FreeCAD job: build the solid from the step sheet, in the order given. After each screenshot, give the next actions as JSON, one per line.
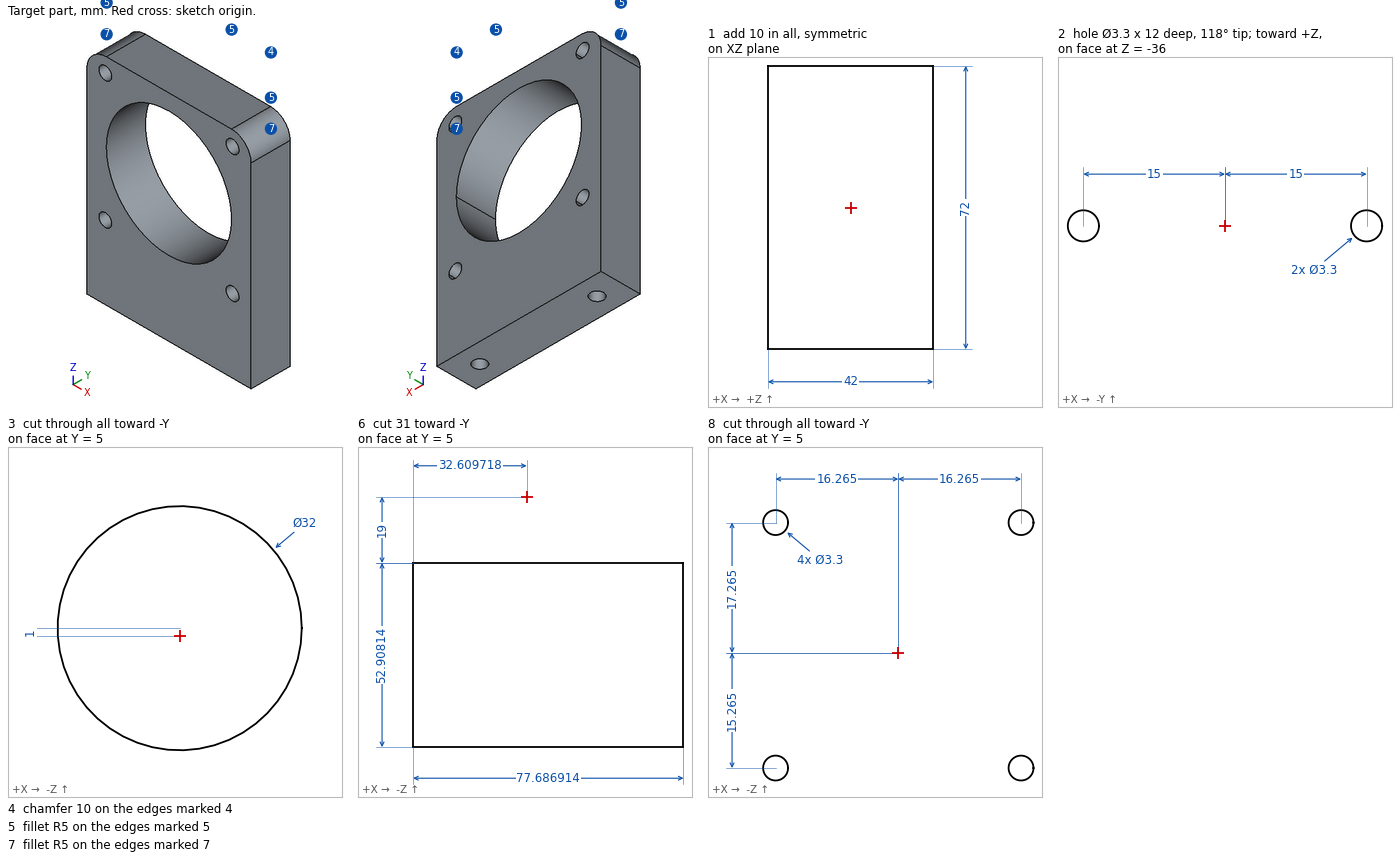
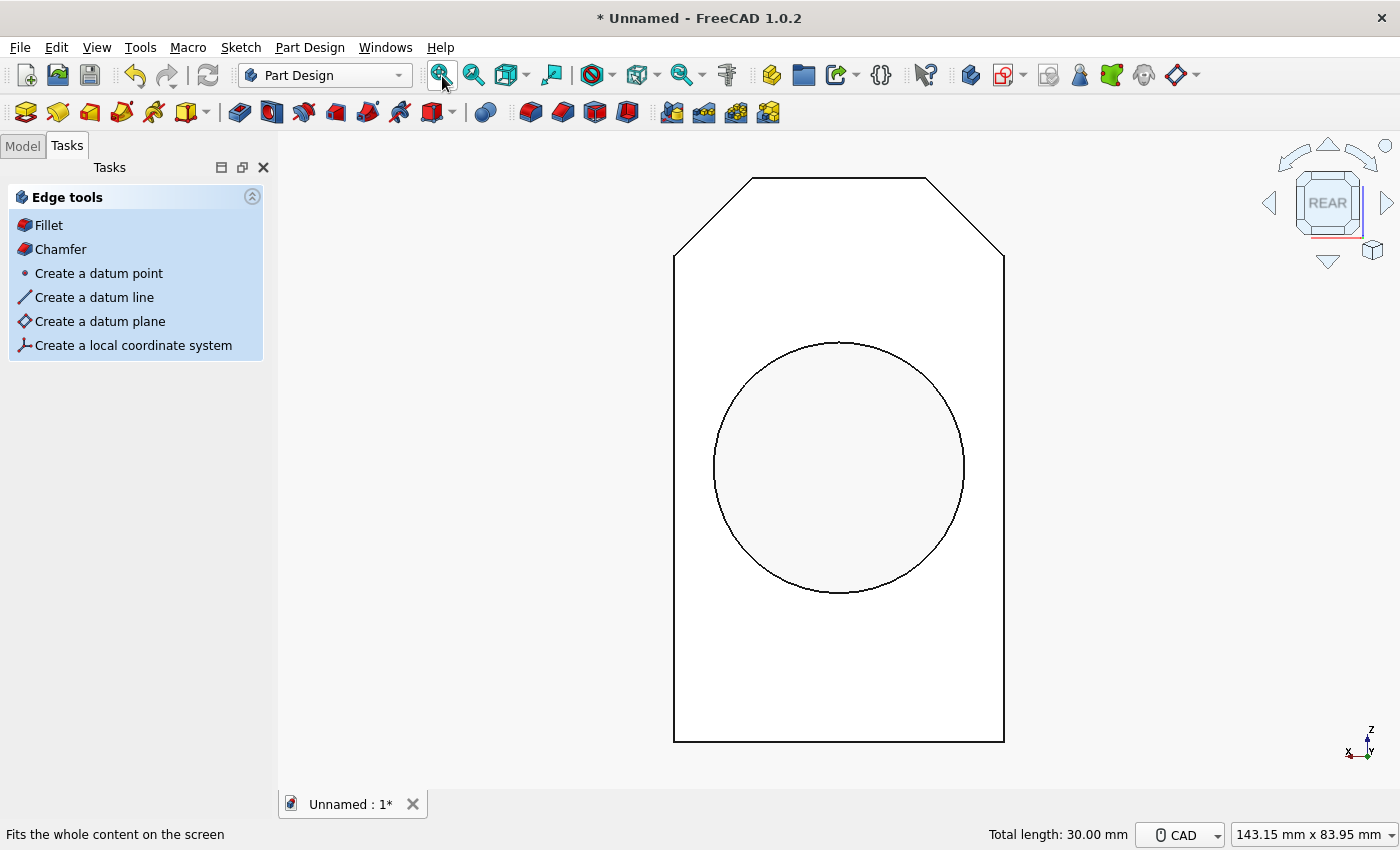
{"action": "key", "text": "6"}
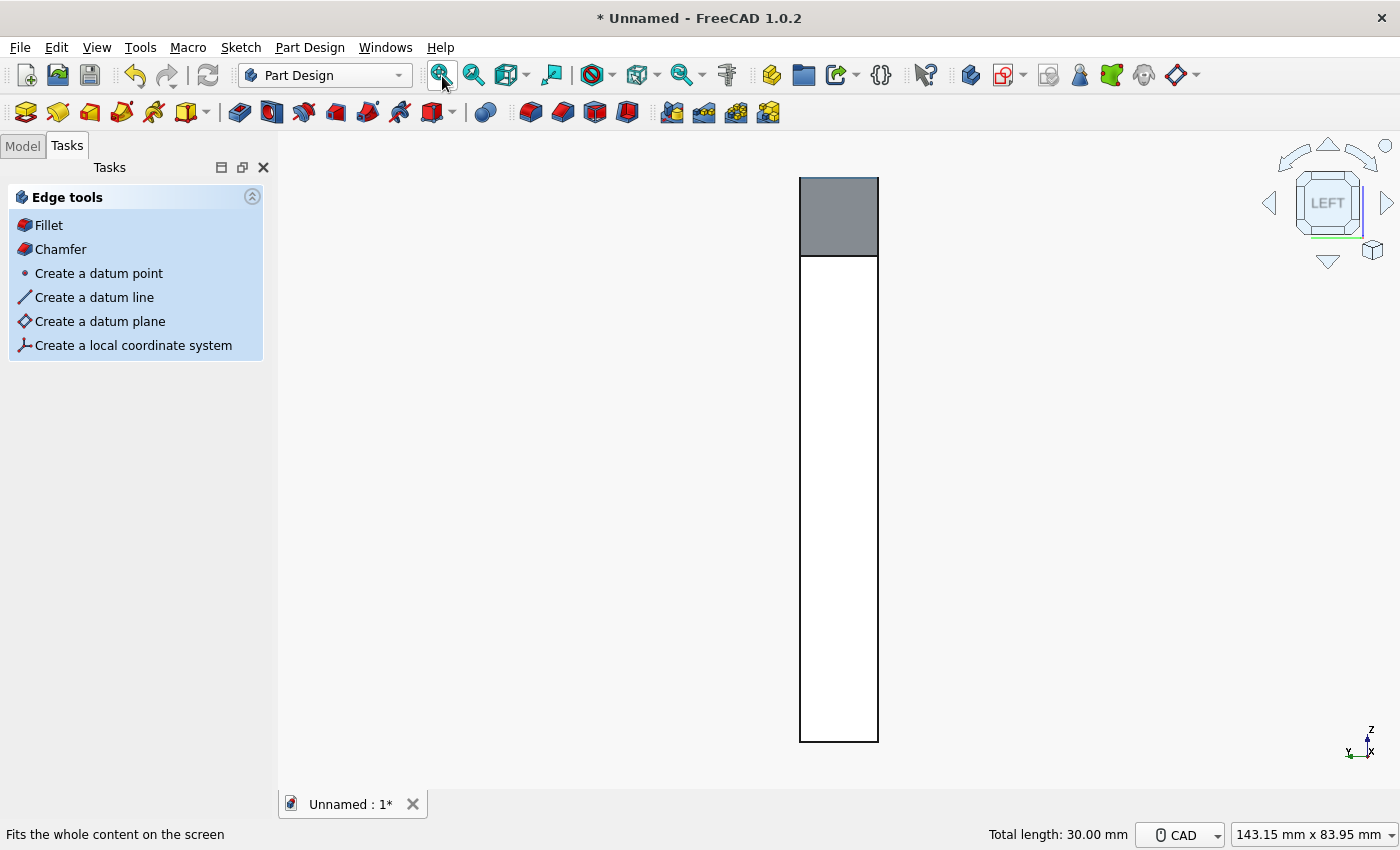
{"action": "left_click", "coordinate": [839, 255], "text": "ctrl"}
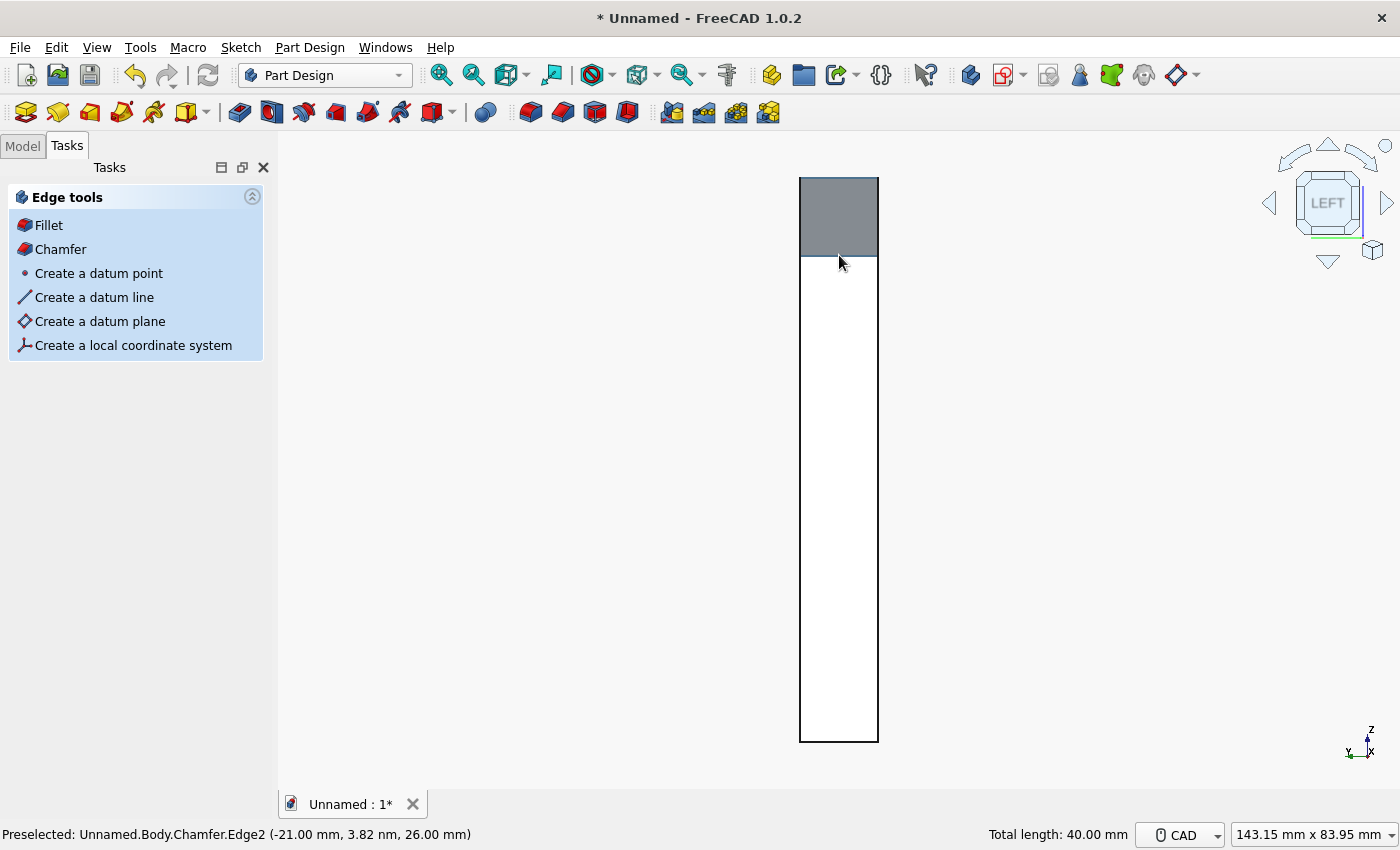
{"action": "left_click", "coordinate": [532, 112]}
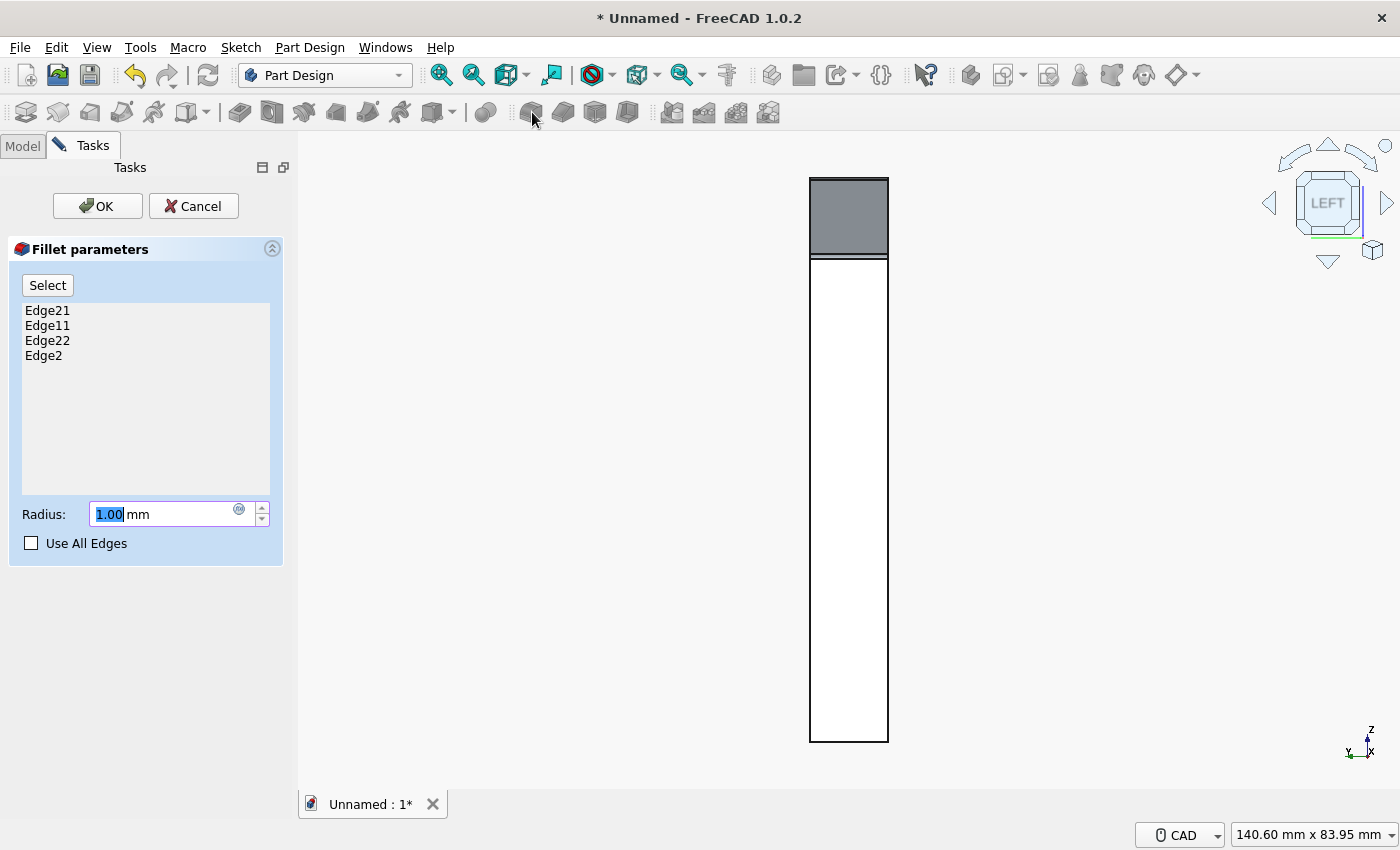
{"action": "type", "text": "5"}
{"action": "key", "text": "Tab"}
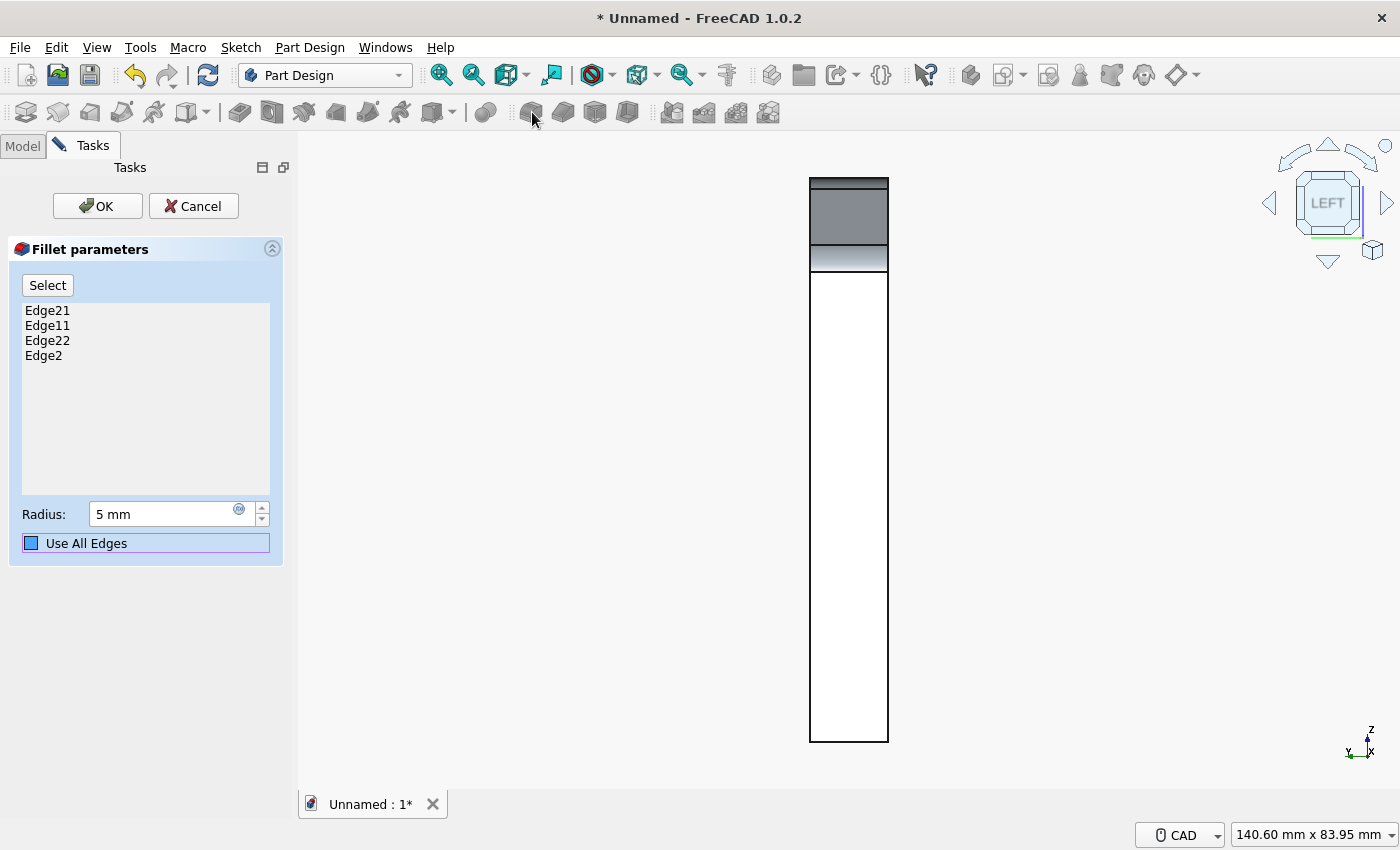
{"action": "left_click", "coordinate": [98, 206]}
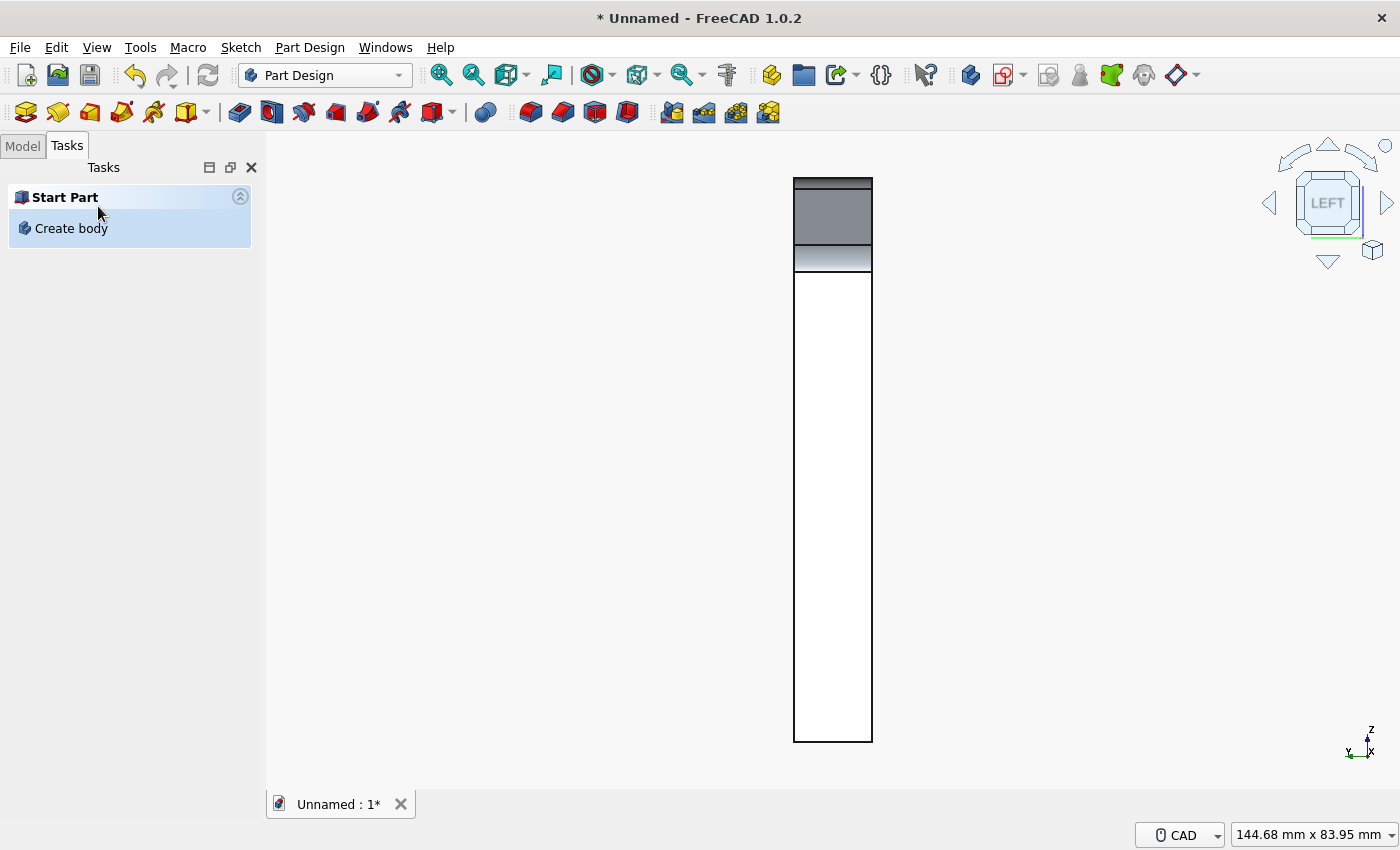
{"action": "key", "text": "4"}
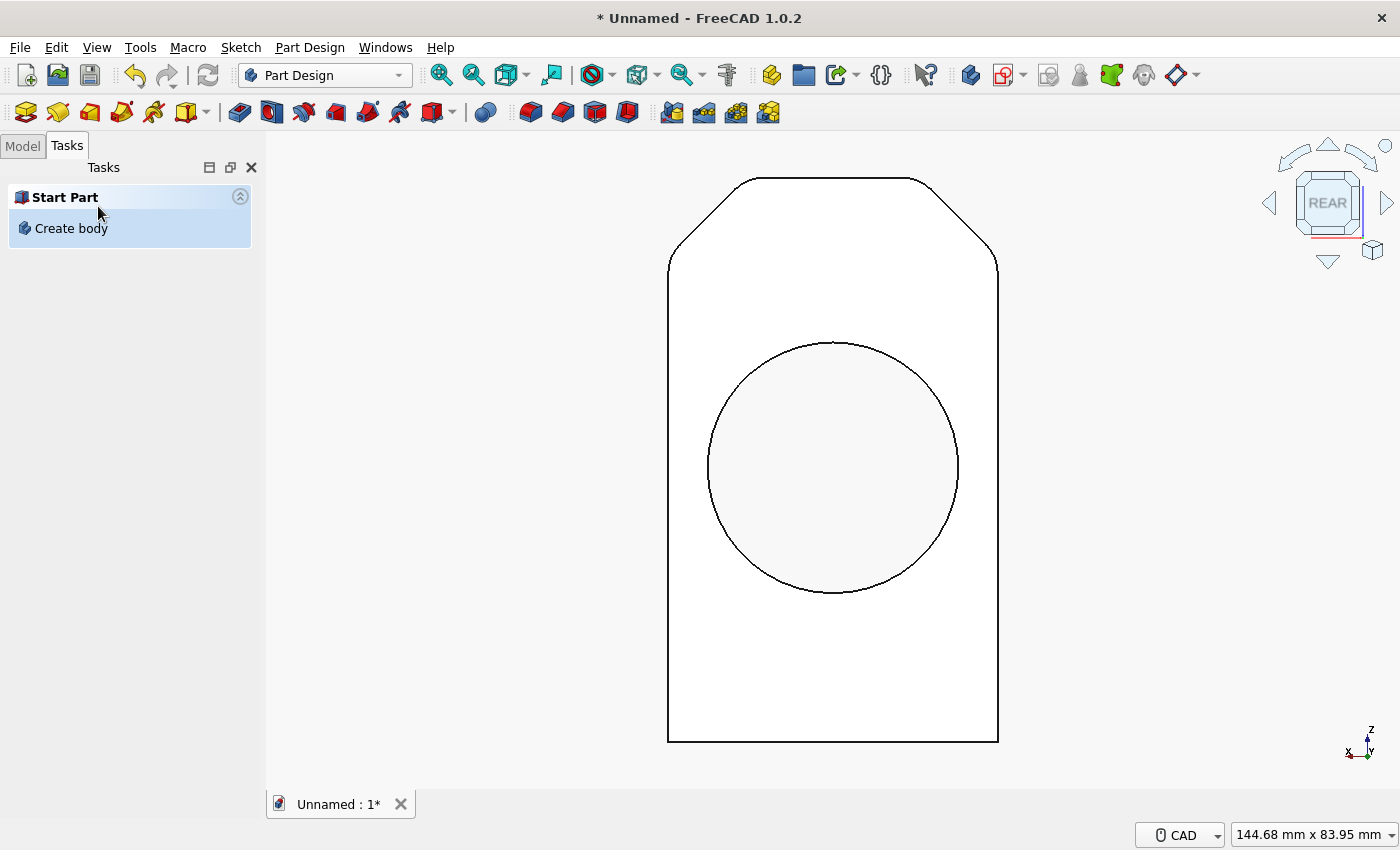
{"action": "left_click", "coordinate": [927, 298]}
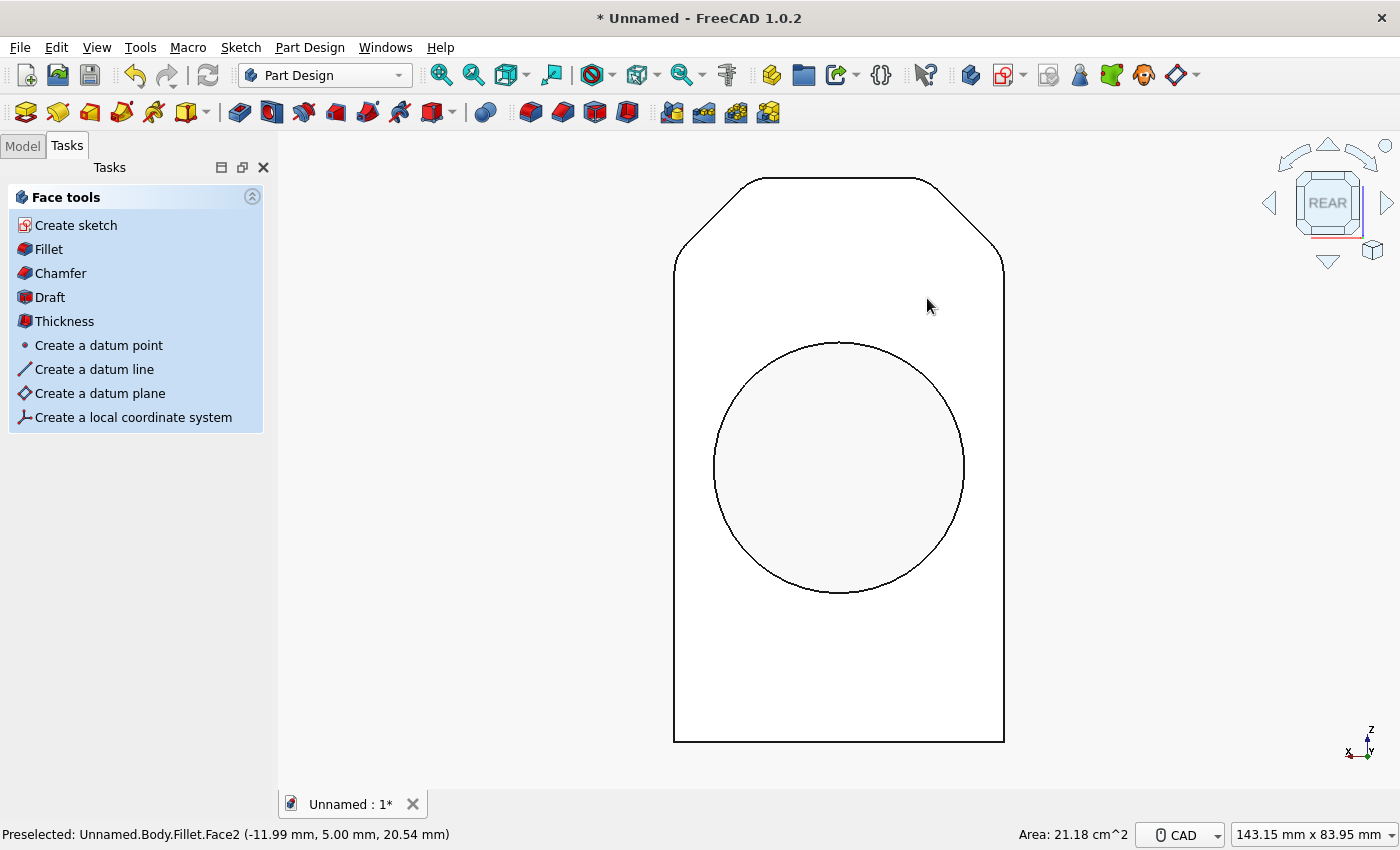
{"action": "left_click", "coordinate": [1004, 76]}